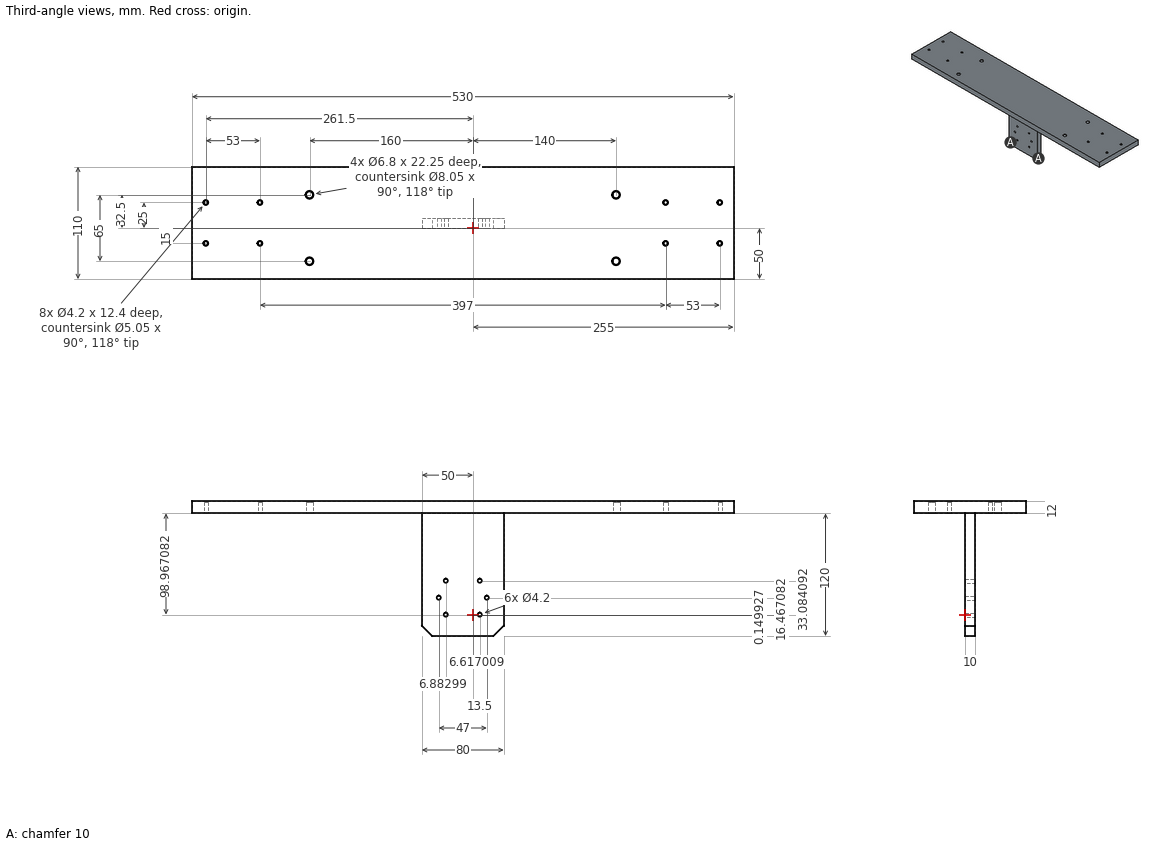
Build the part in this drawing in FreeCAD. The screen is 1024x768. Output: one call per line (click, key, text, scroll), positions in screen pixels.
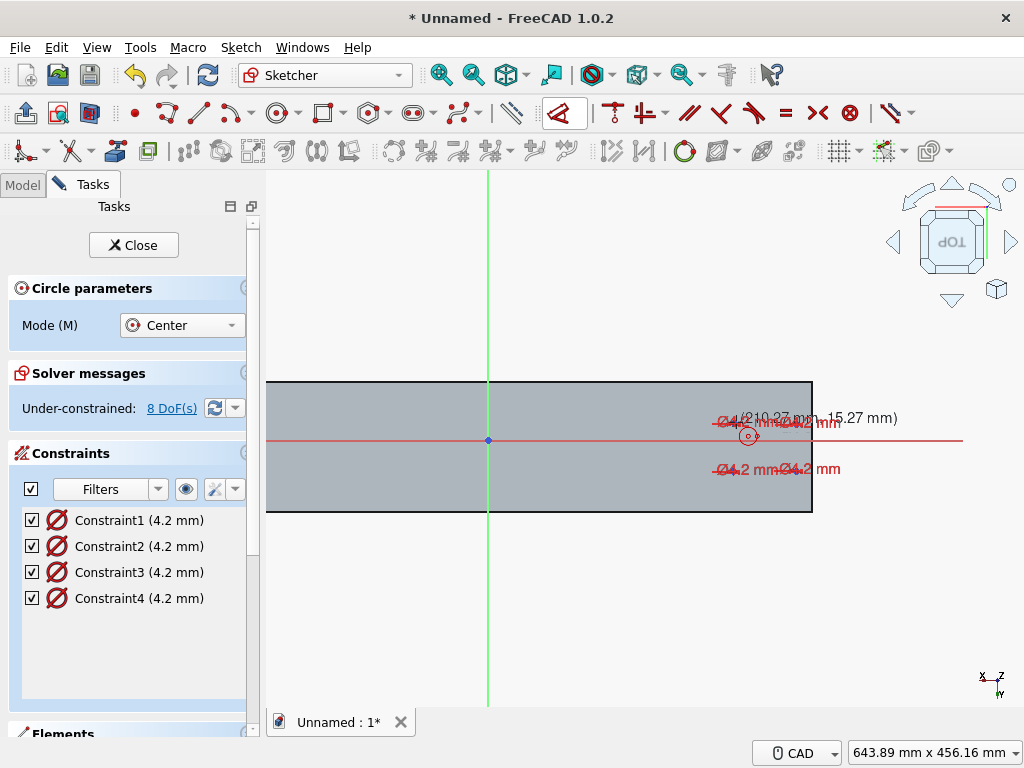
scroll(732, 421, down, 2)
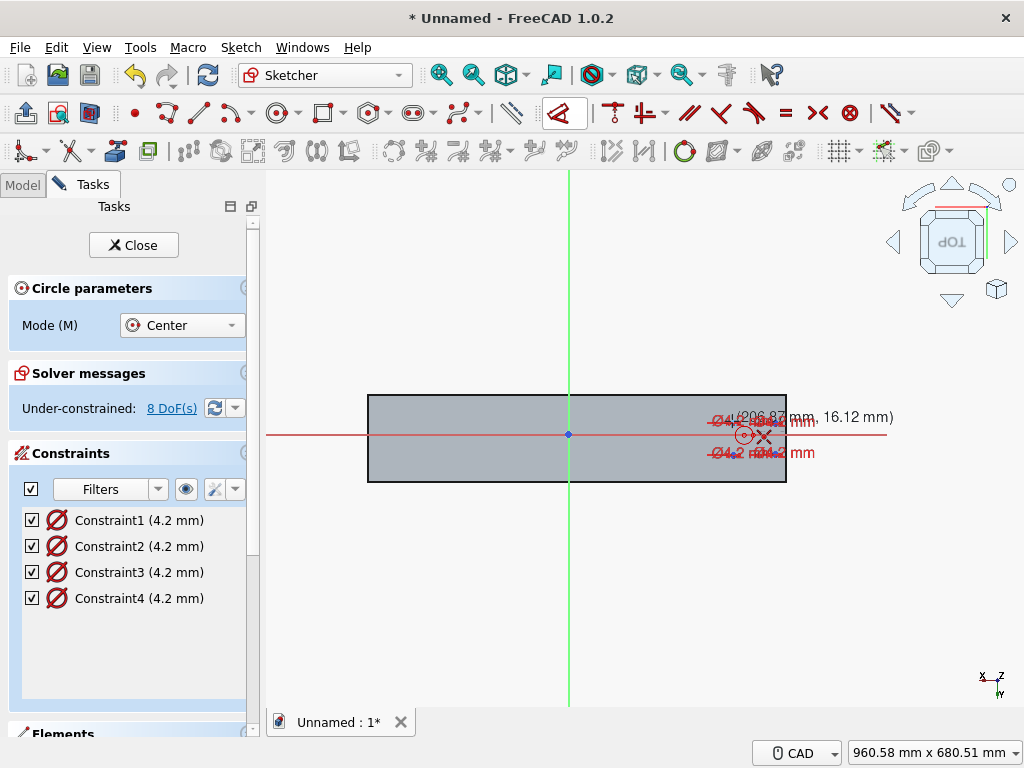
scroll(420, 423, up, 14)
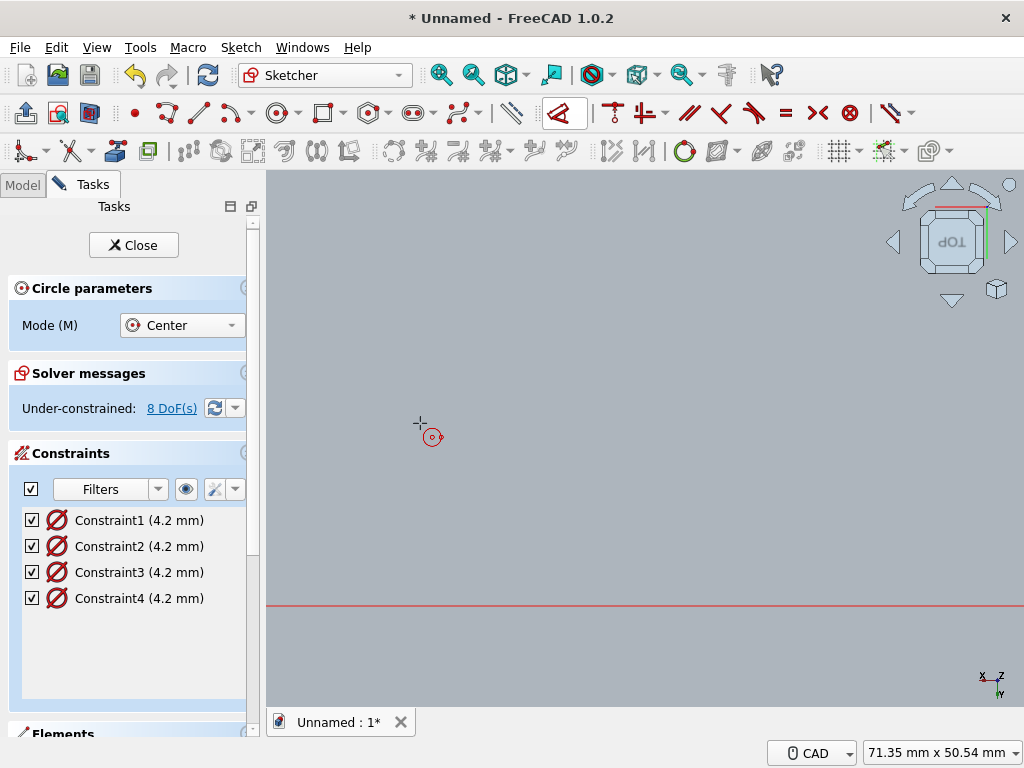
scroll(420, 423, down, 14)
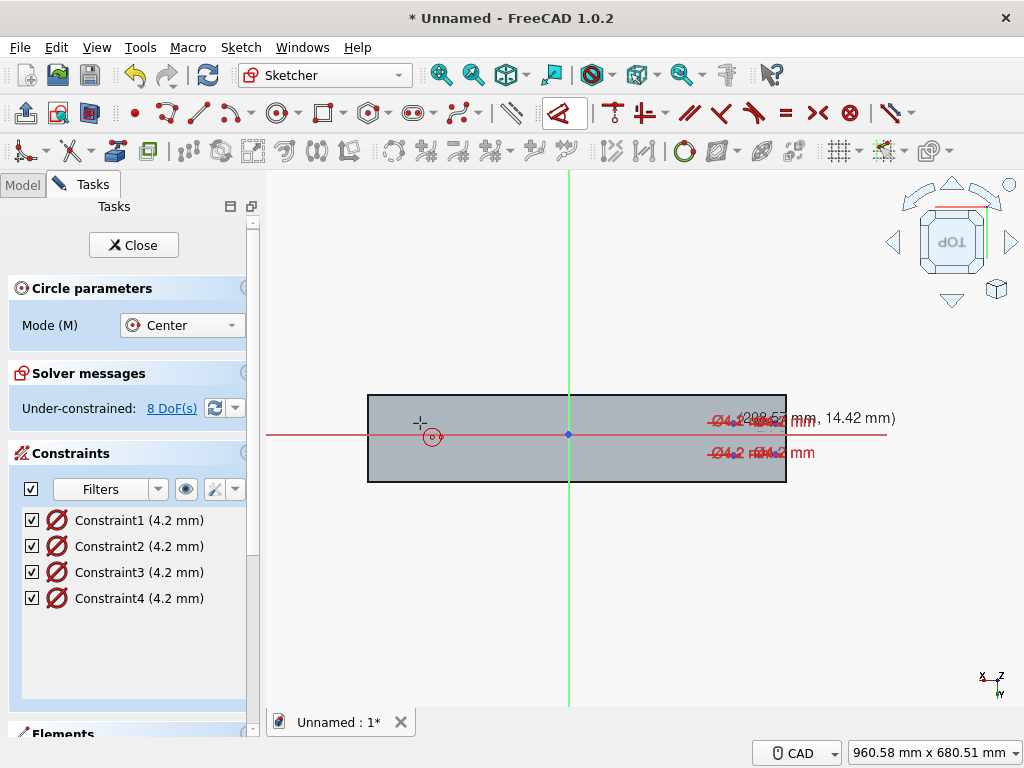
scroll(420, 423, up, 2)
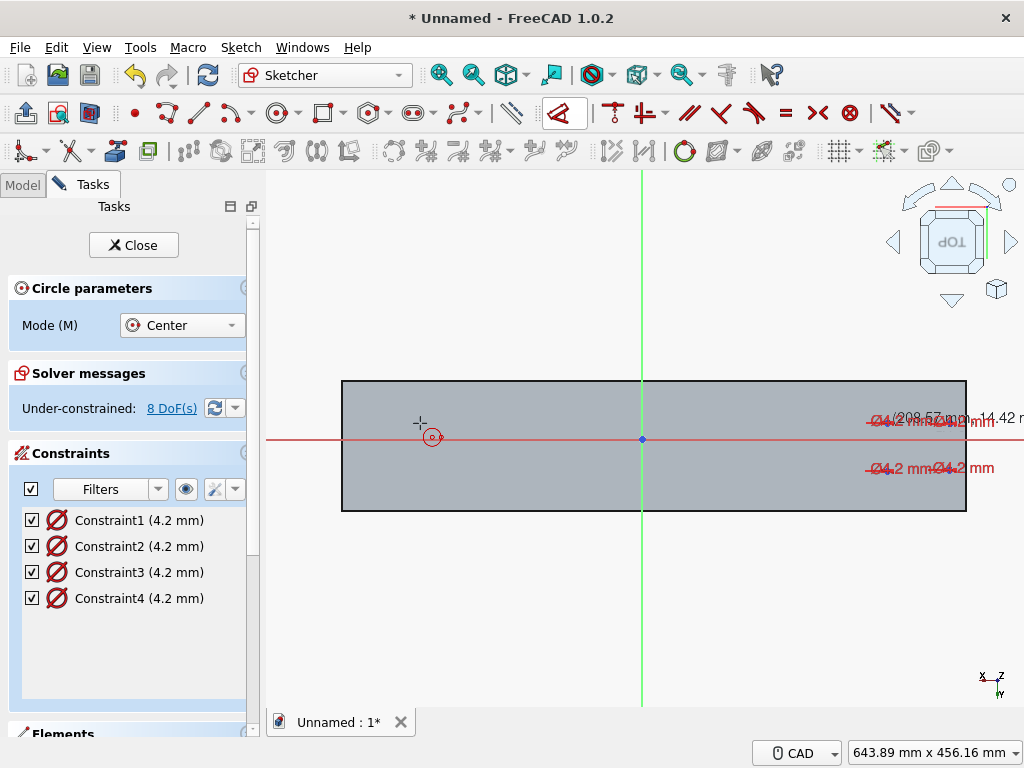
click(420, 422)
move(422, 421)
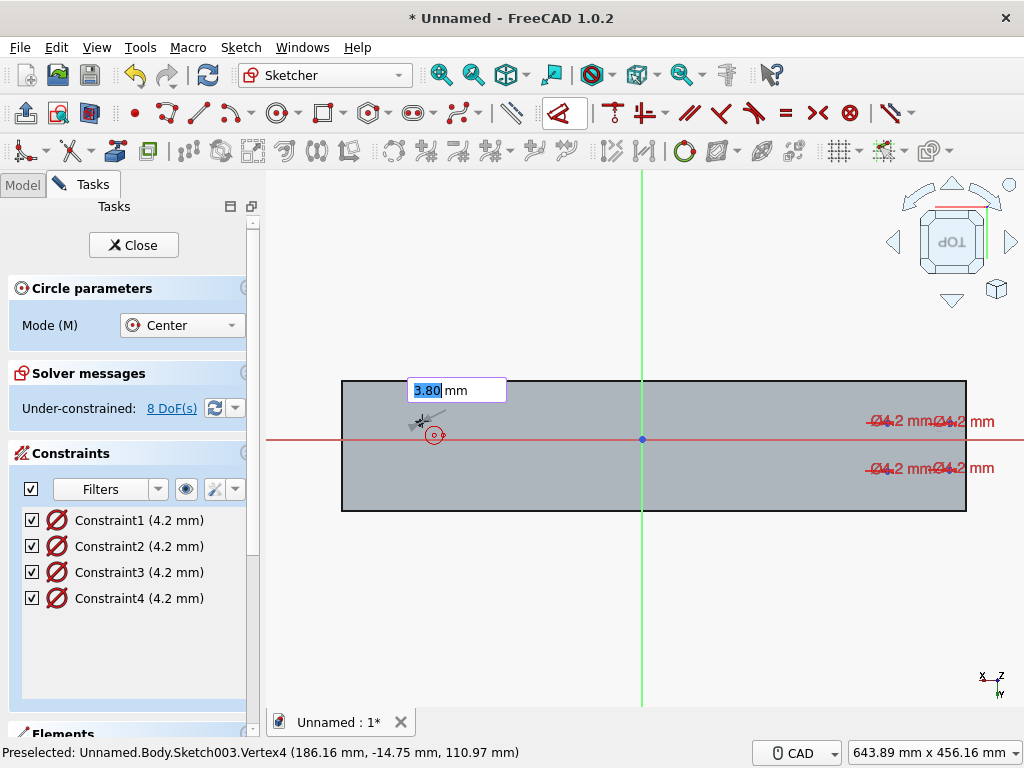
text(4.2)
key(Return)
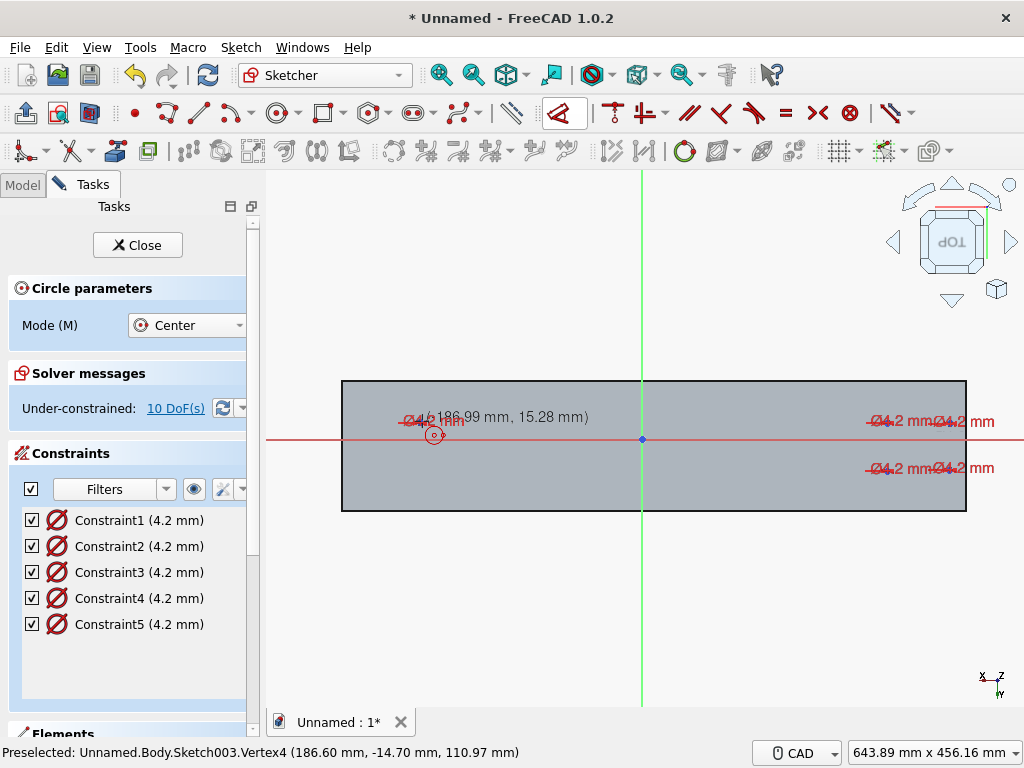
scroll(420, 469, up, 12)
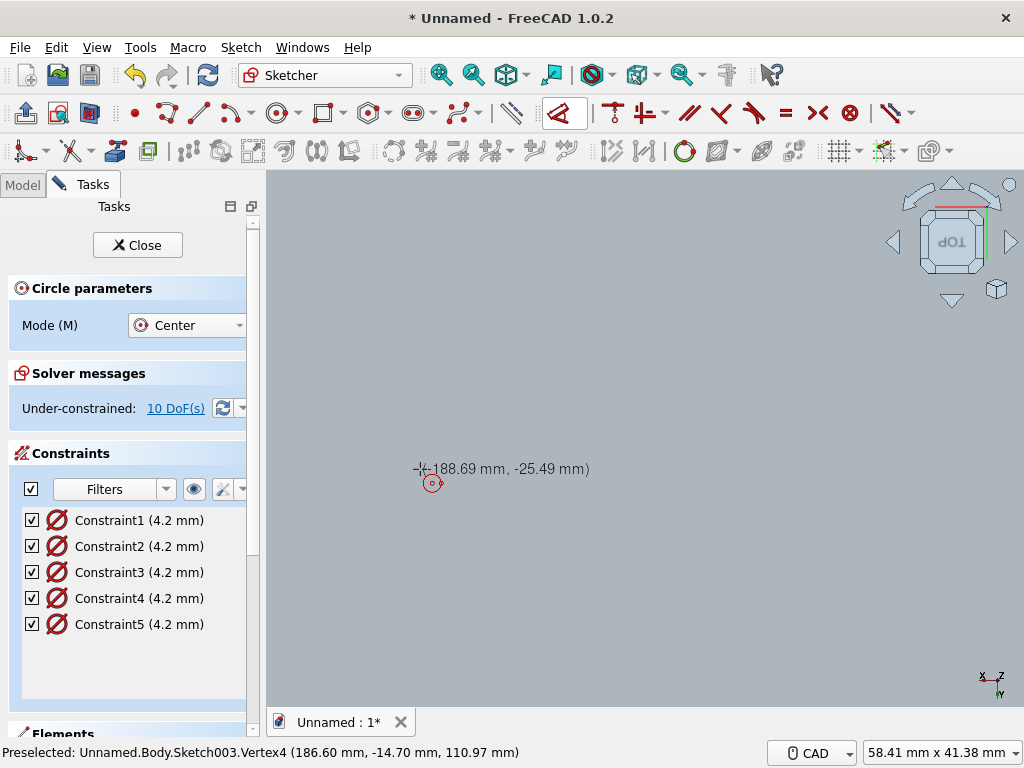
scroll(420, 453, down, 14)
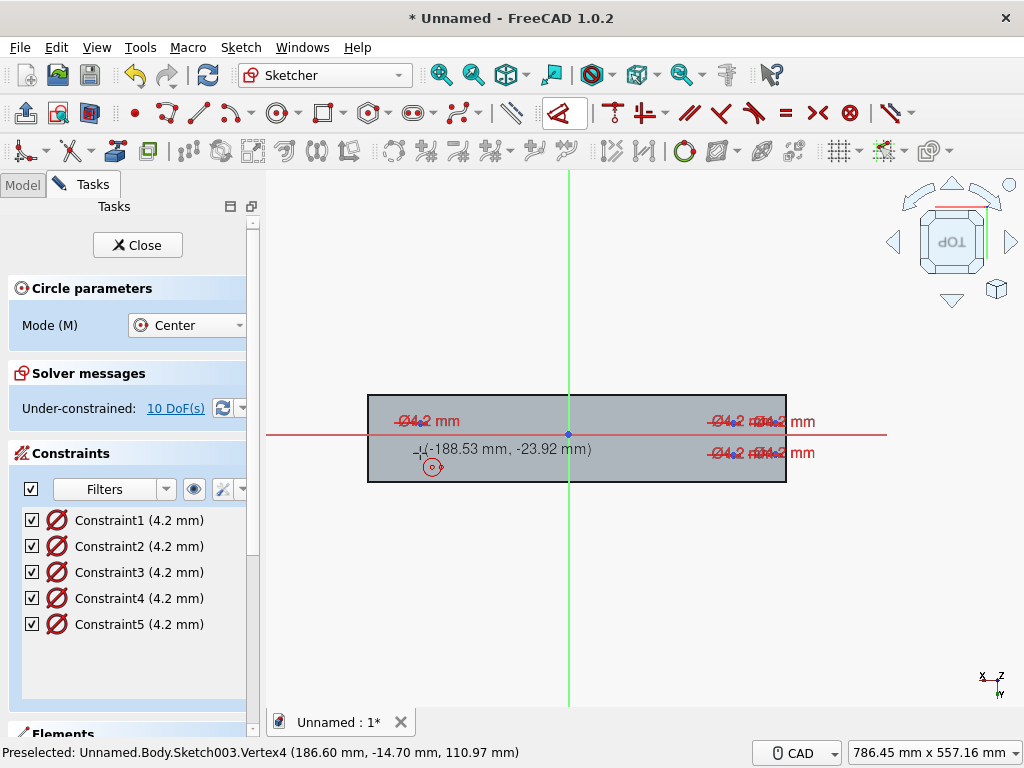
click(420, 454)
move(421, 453)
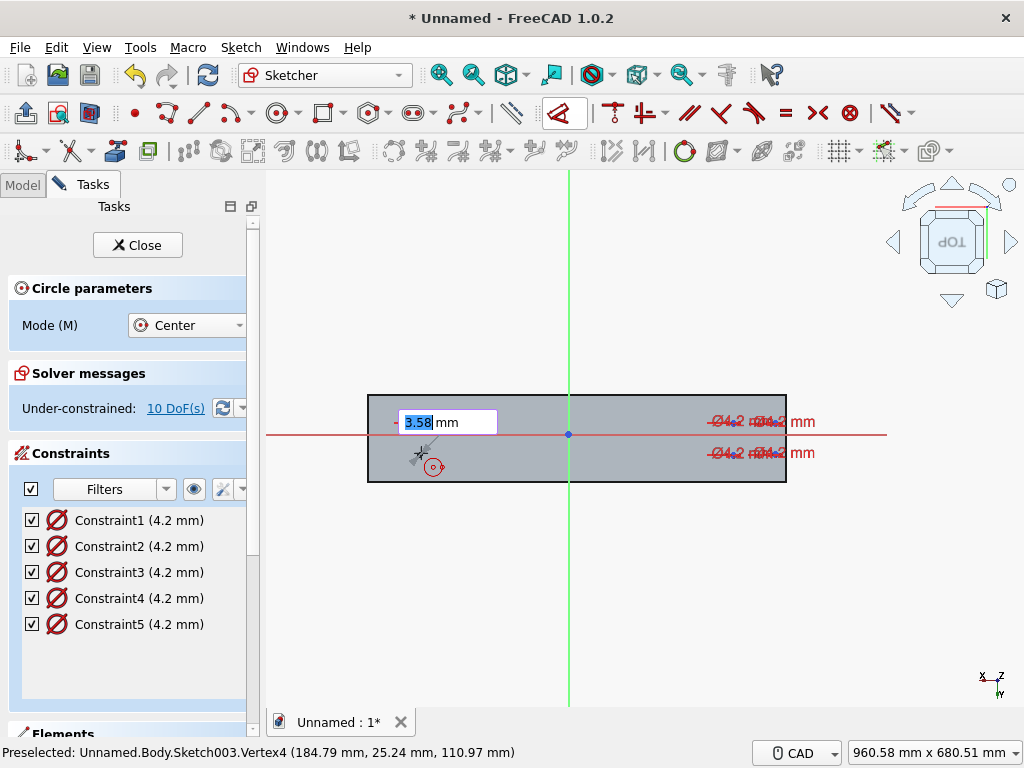
text(4.2)
key(Return)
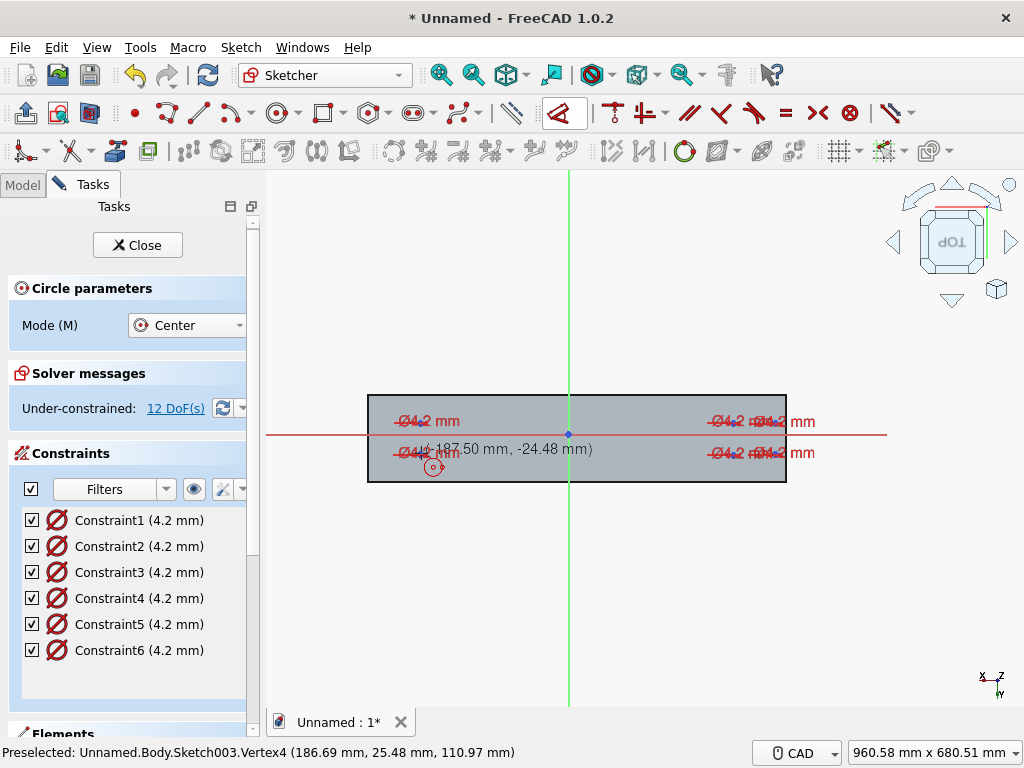
scroll(378, 423, up, 14)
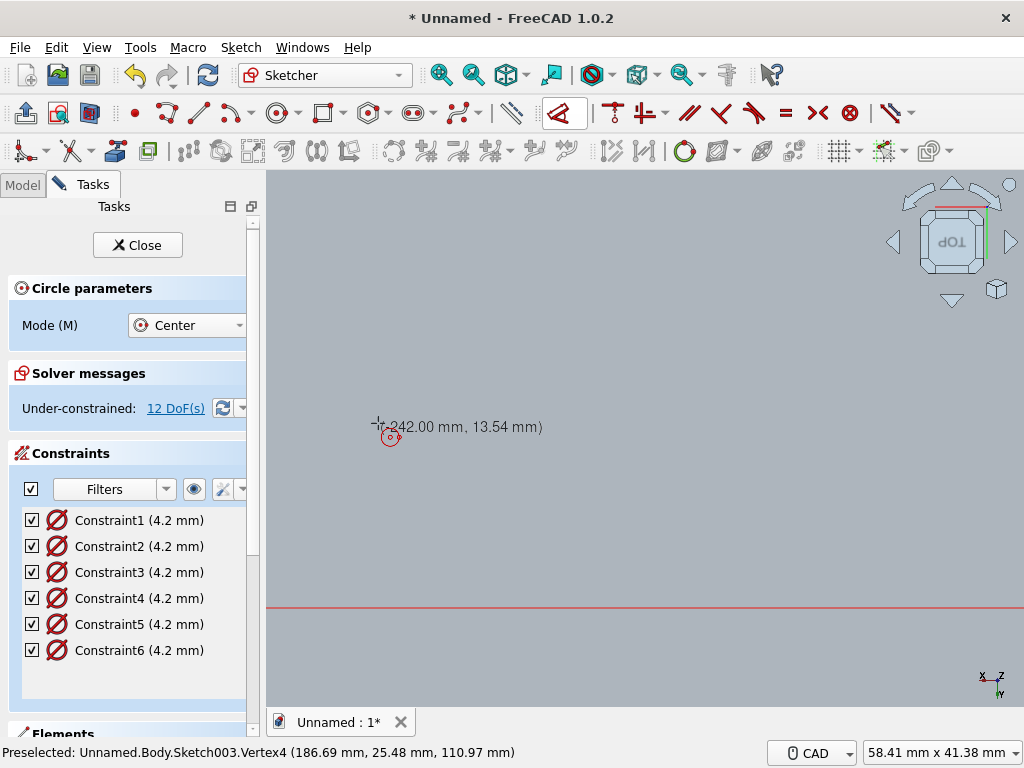
scroll(378, 423, down, 14)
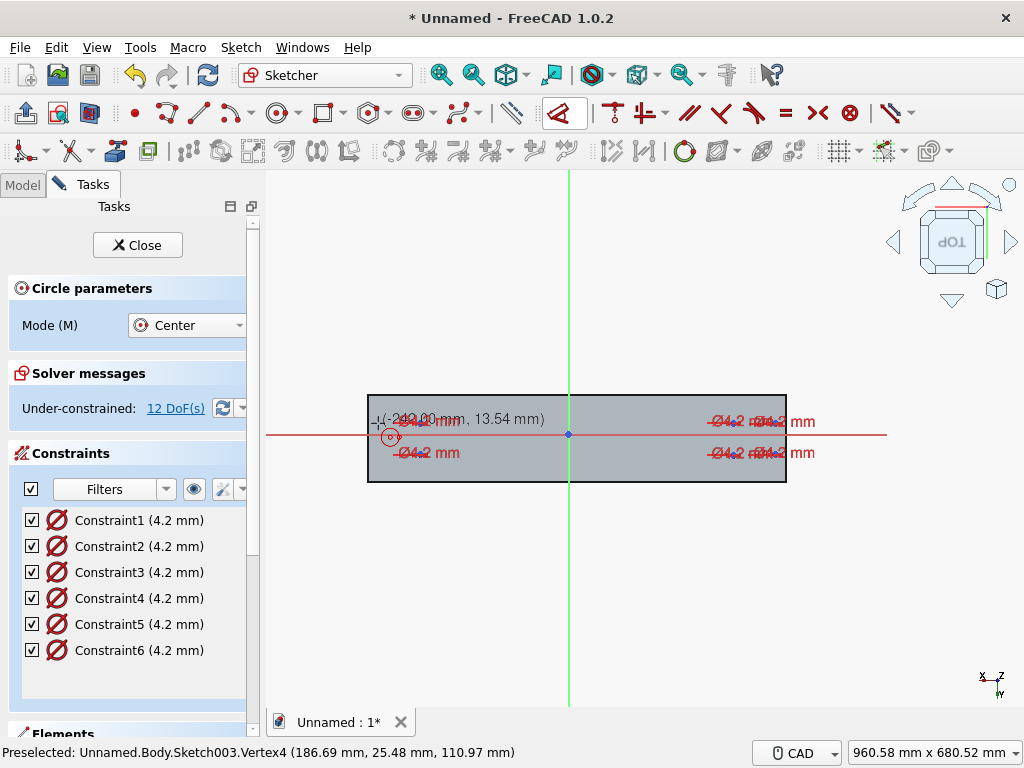
scroll(378, 423, up, 2)